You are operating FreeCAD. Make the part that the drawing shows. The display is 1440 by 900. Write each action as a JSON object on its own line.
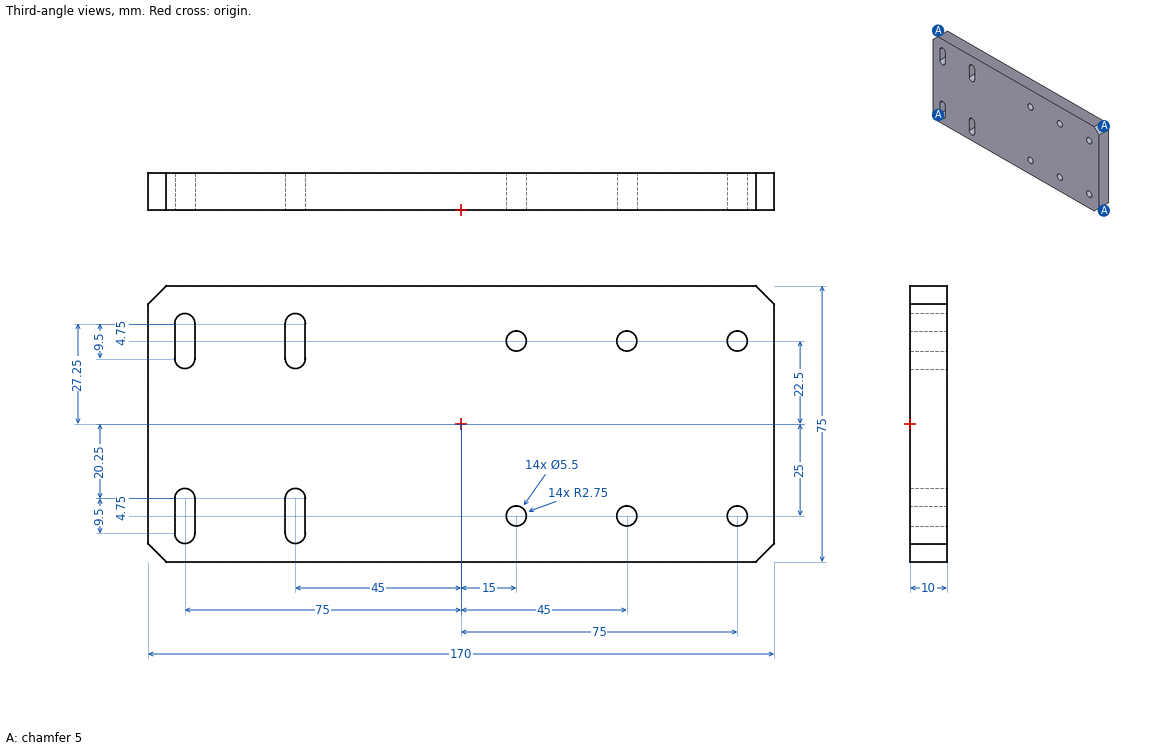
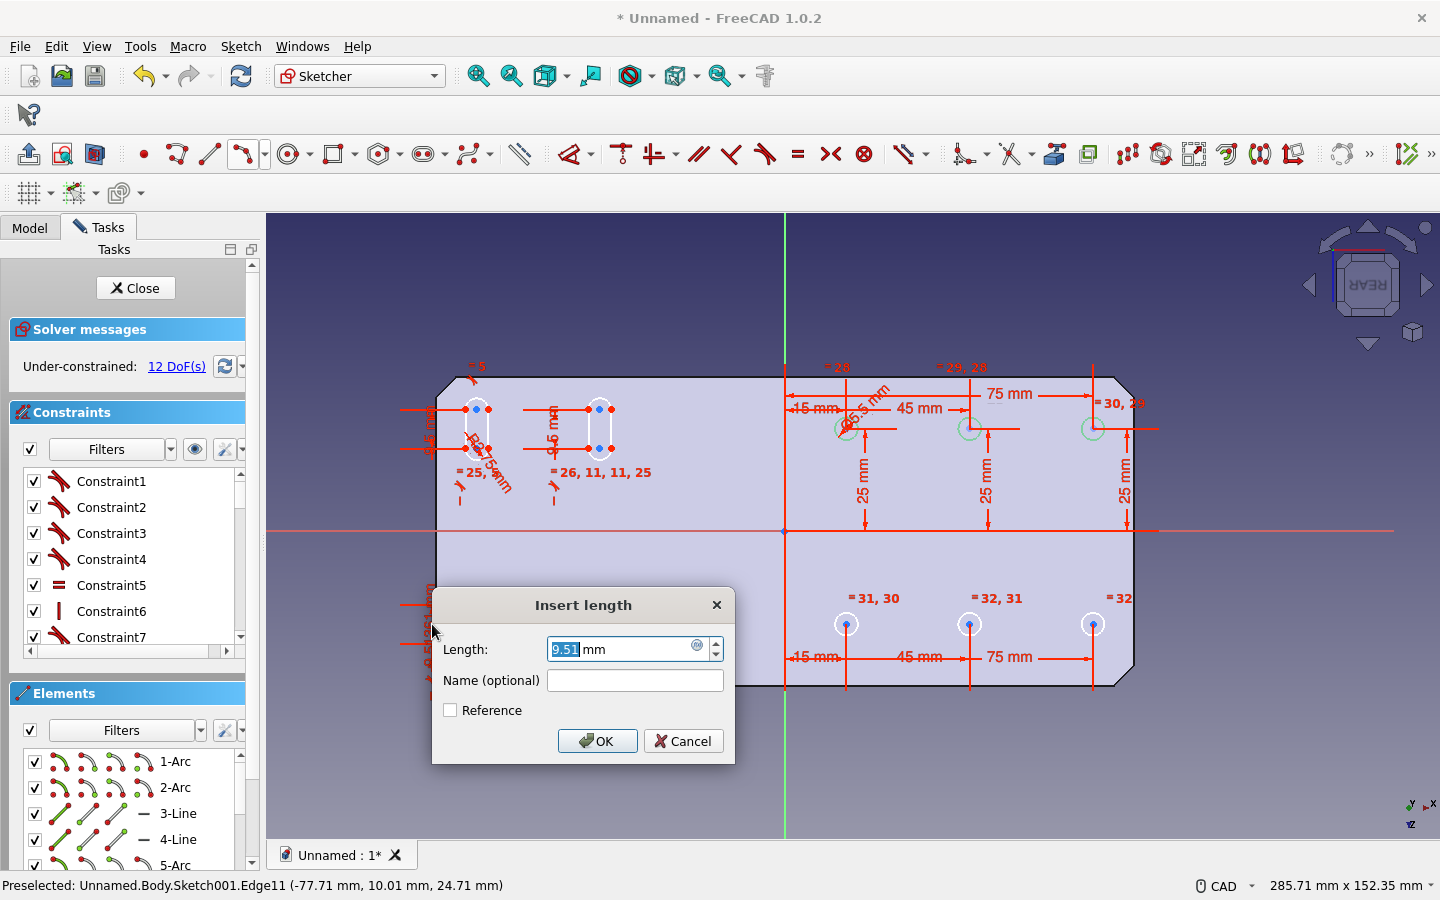
{"action": "type", "text": "9.5"}
{"action": "key", "text": "Return"}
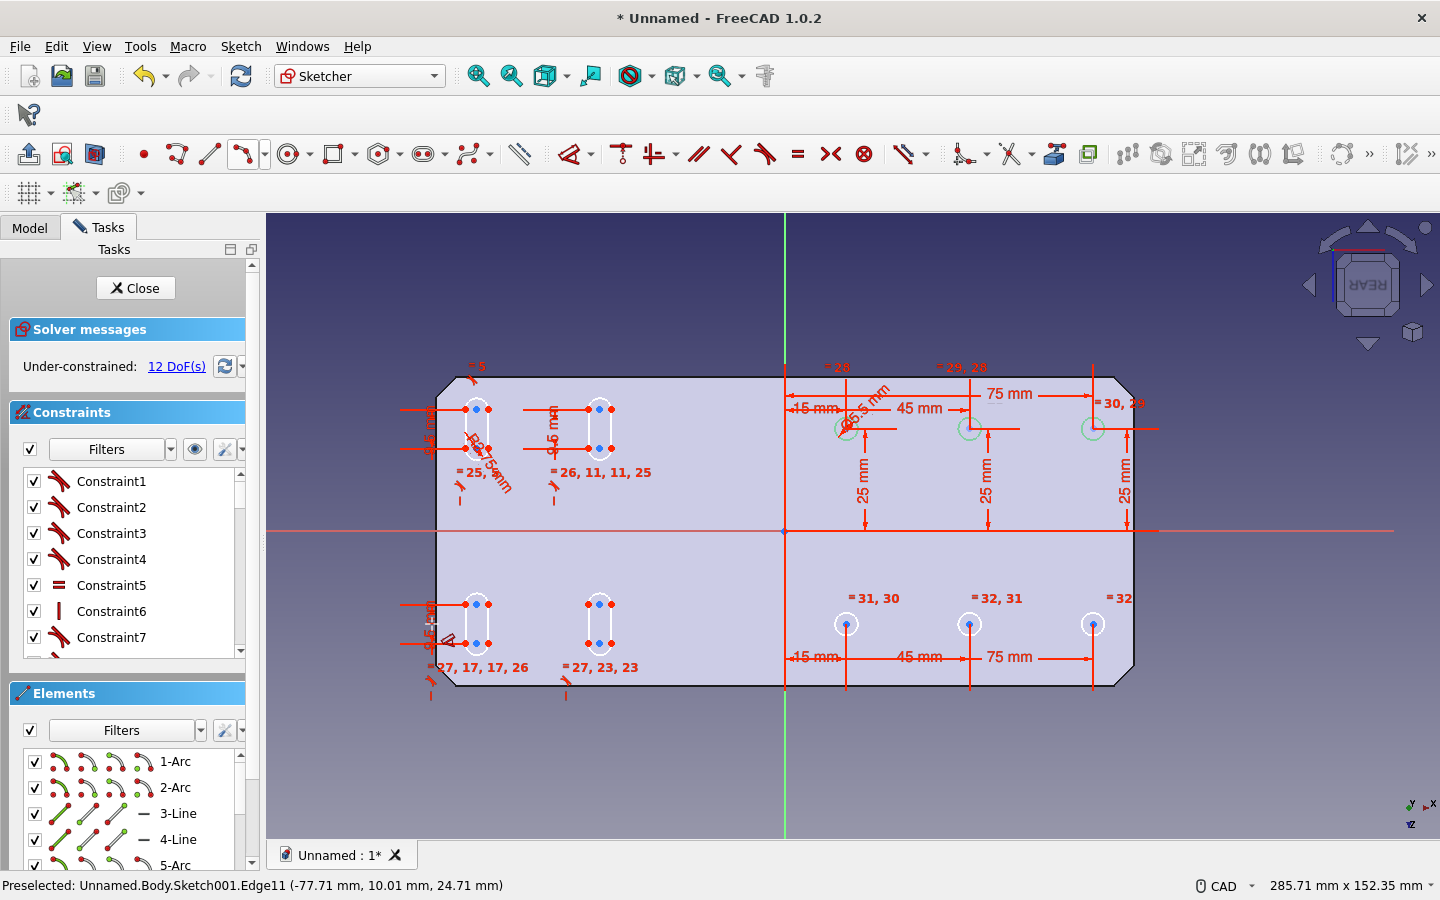
{"action": "left_click", "coordinate": [589, 632]}
{"action": "left_click", "coordinate": [555, 624]}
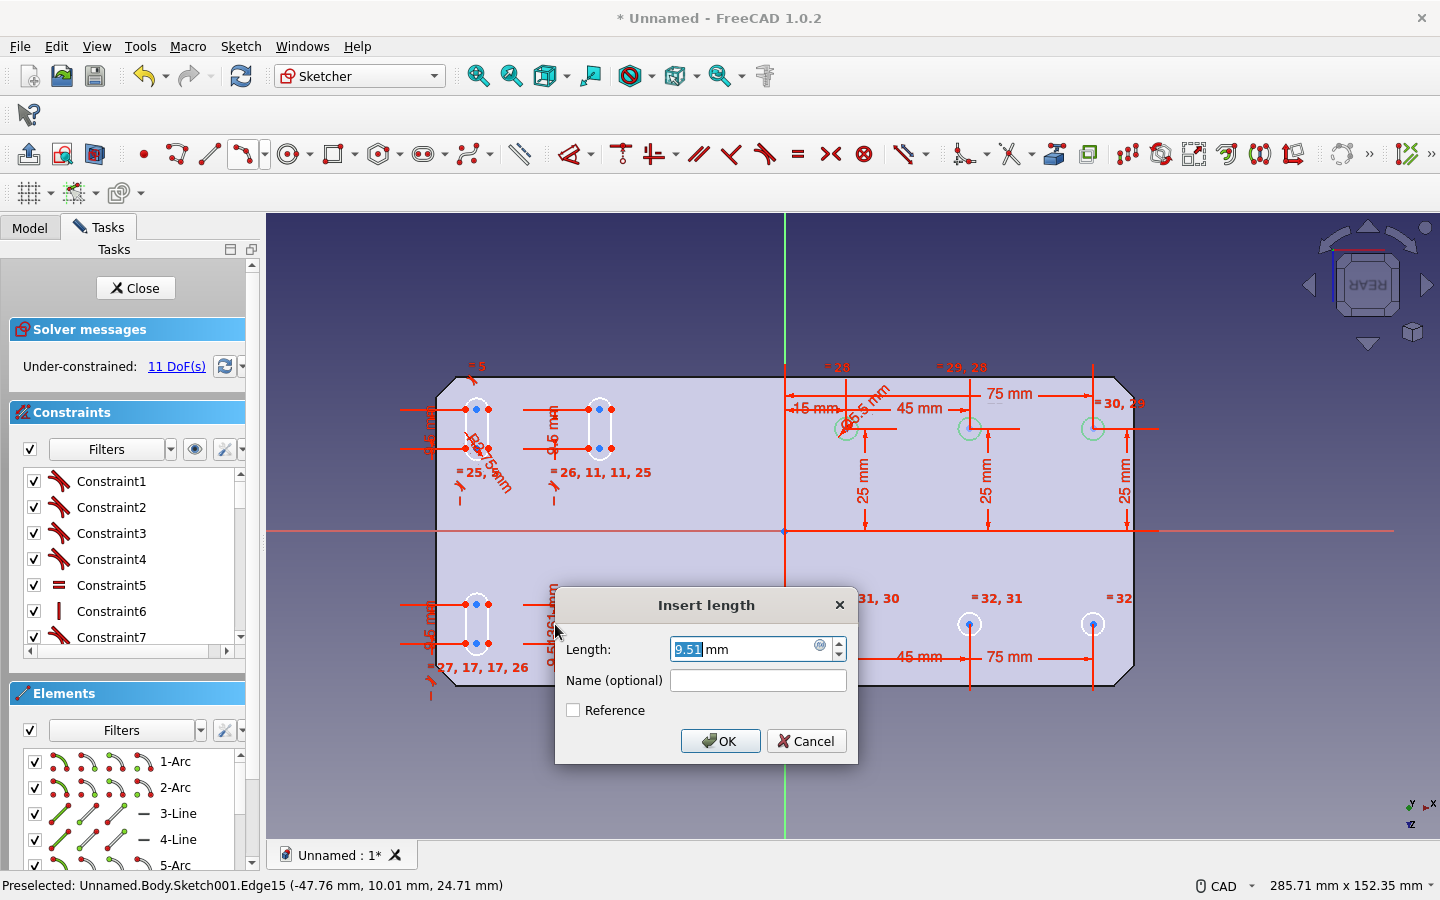
{"action": "type", "text": "9.5"}
{"action": "key", "text": "Return"}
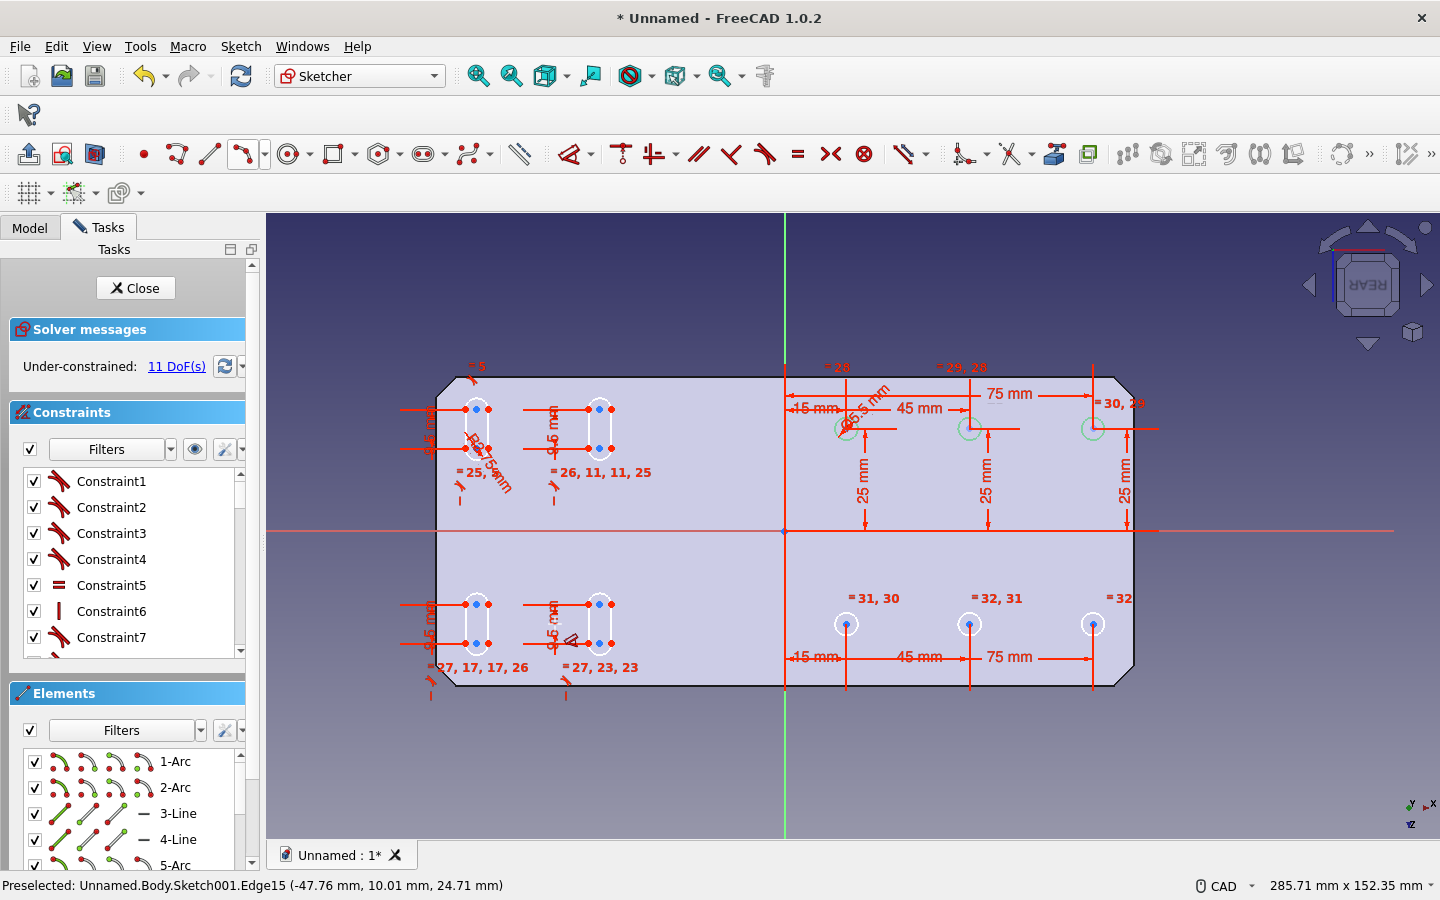
{"action": "left_click", "coordinate": [477, 449]}
{"action": "left_click", "coordinate": [631, 415]}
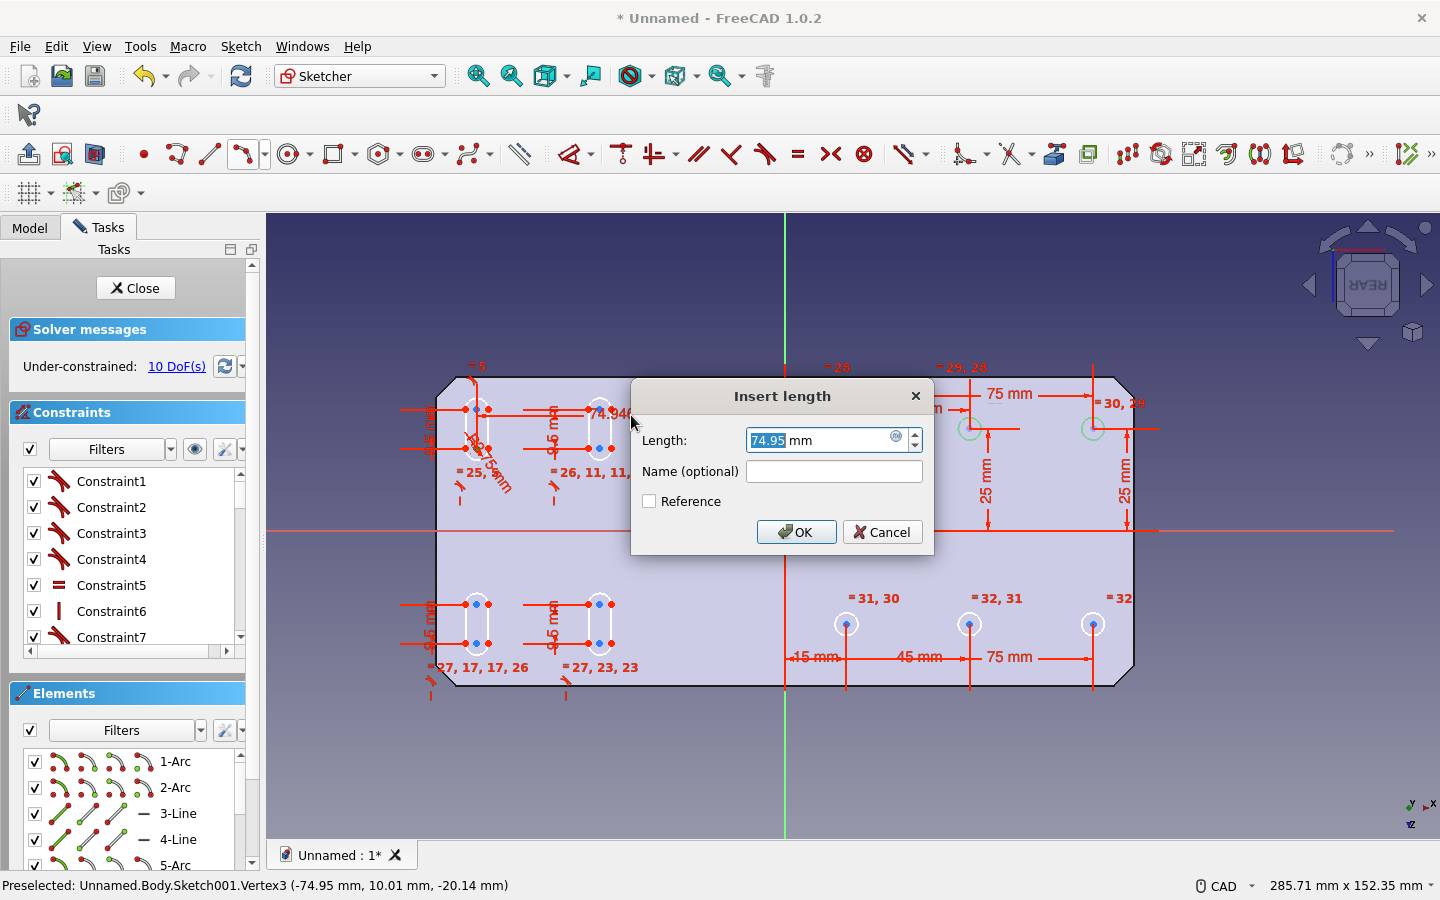
{"action": "type", "text": "75"}
{"action": "key", "text": "Return"}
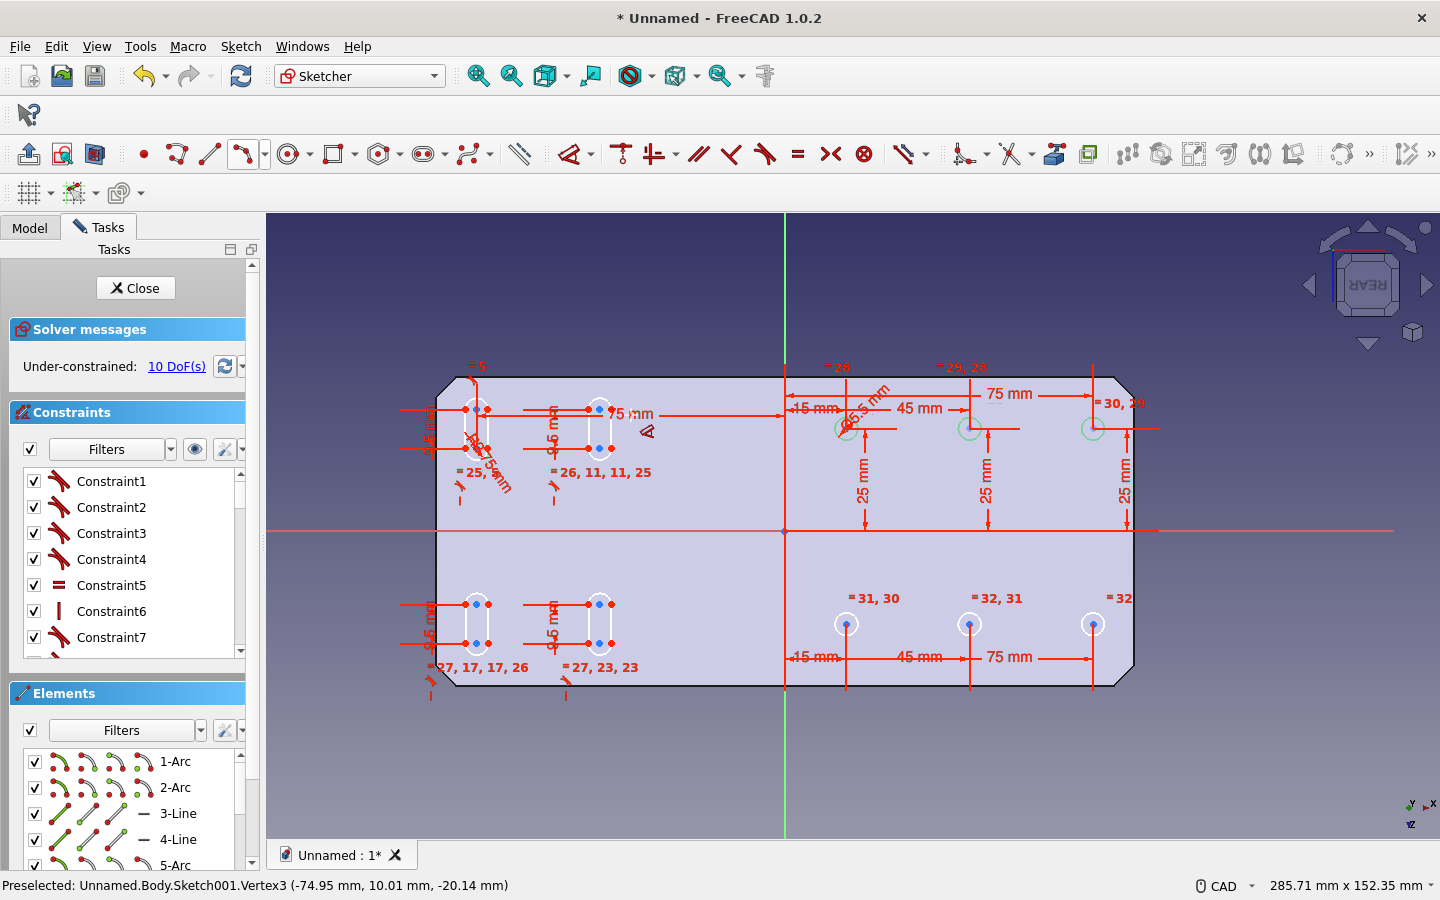
{"action": "left_click", "coordinate": [600, 449]}
{"action": "left_click", "coordinate": [735, 415]}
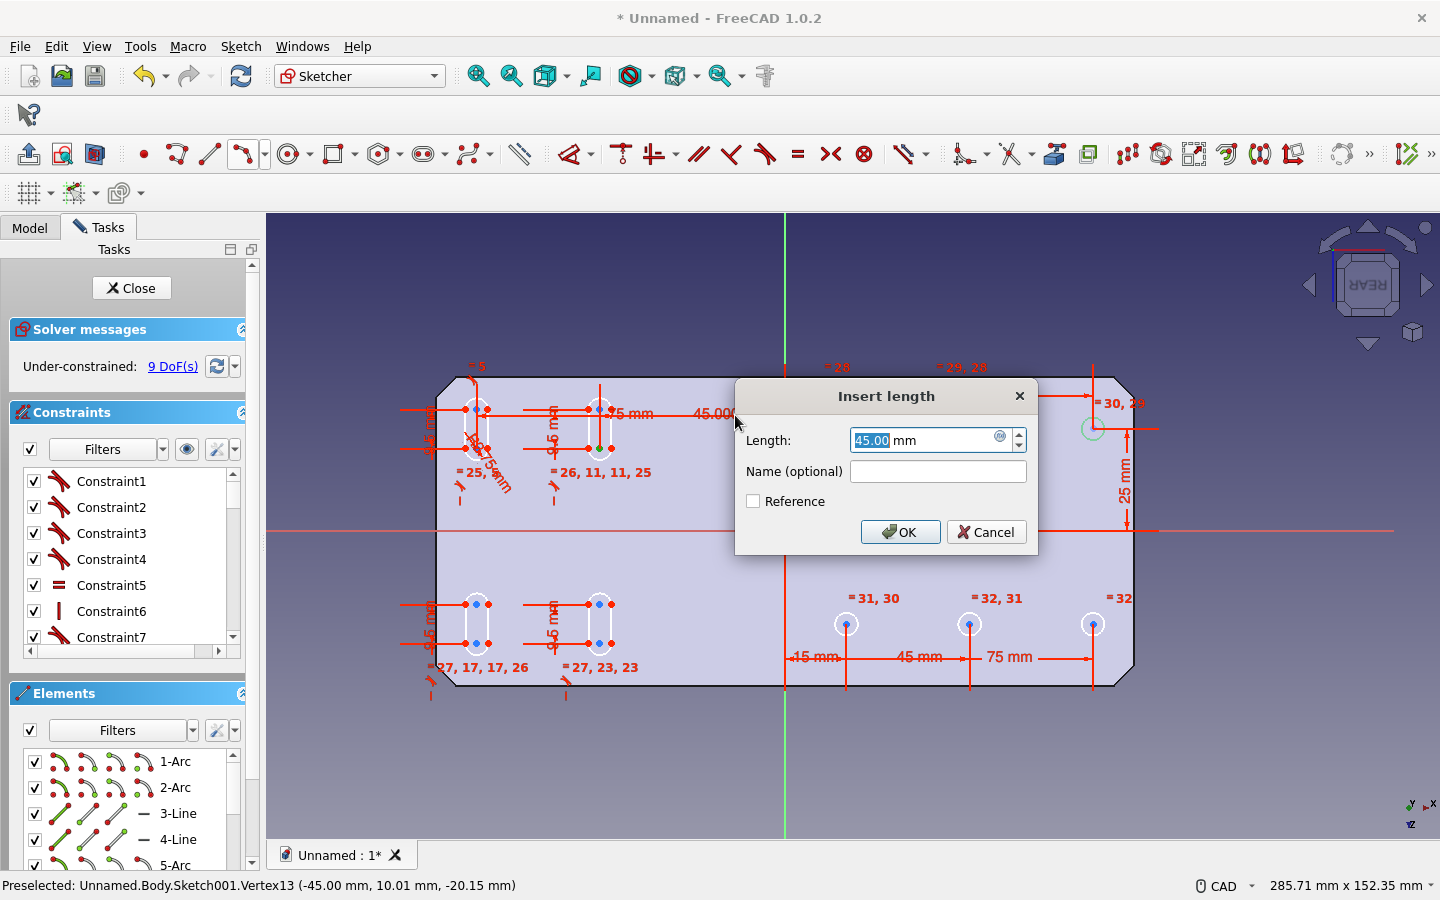
{"action": "type", "text": "45"}
{"action": "key", "text": "Return"}